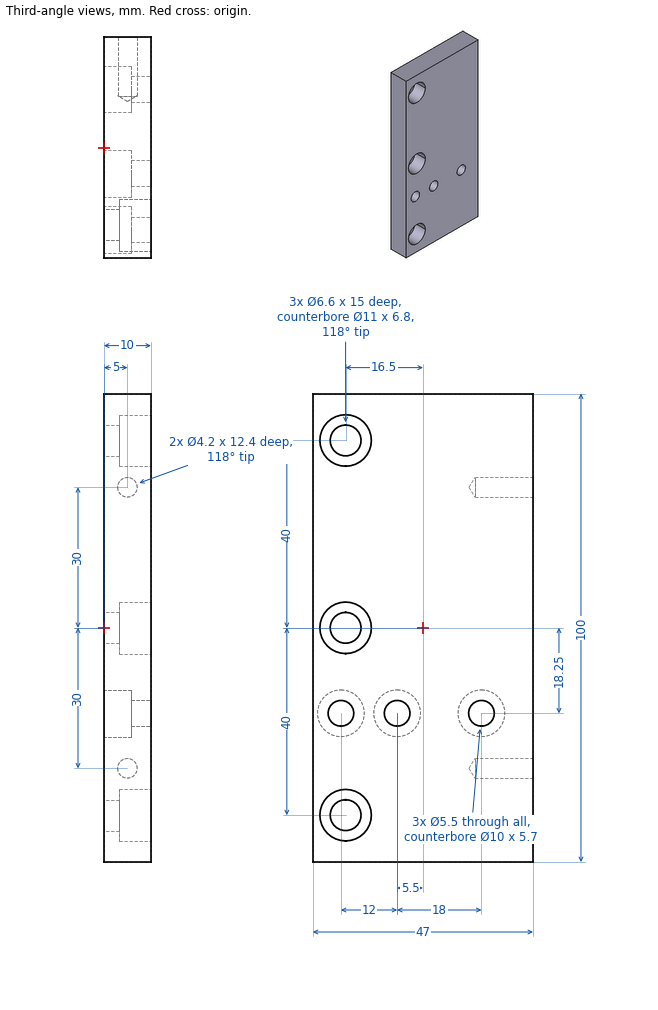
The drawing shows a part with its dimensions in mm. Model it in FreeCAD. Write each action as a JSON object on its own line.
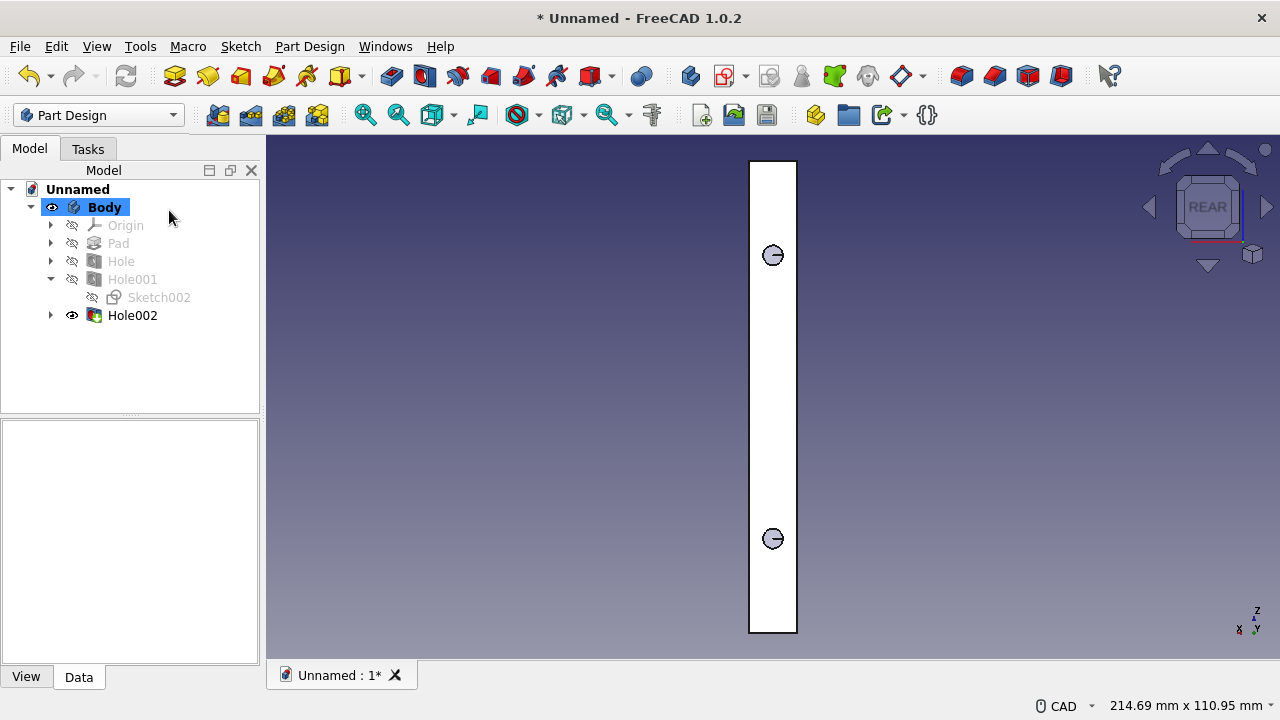
{"action": "key", "text": "0"}